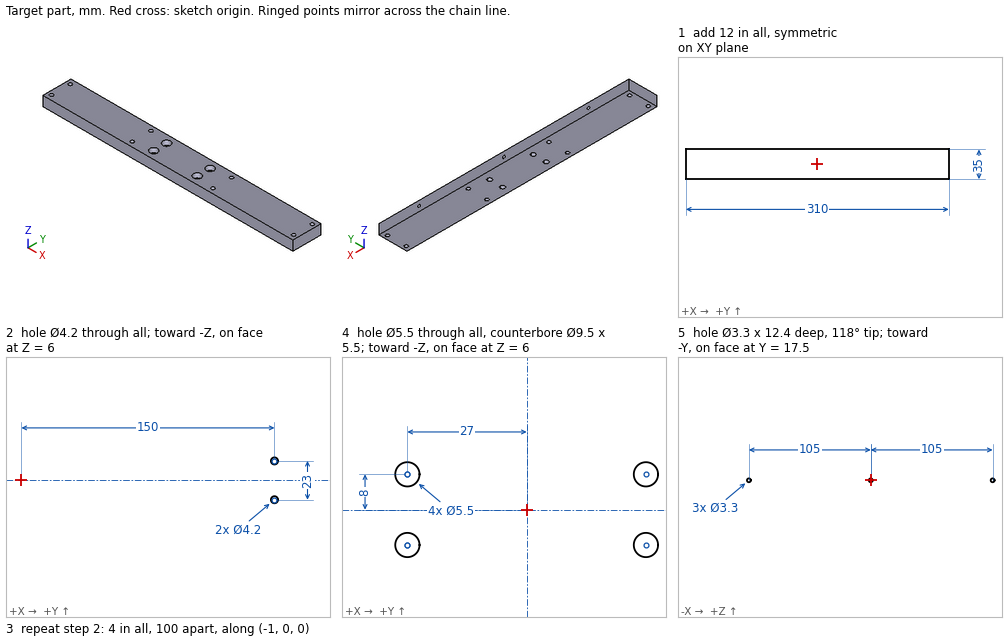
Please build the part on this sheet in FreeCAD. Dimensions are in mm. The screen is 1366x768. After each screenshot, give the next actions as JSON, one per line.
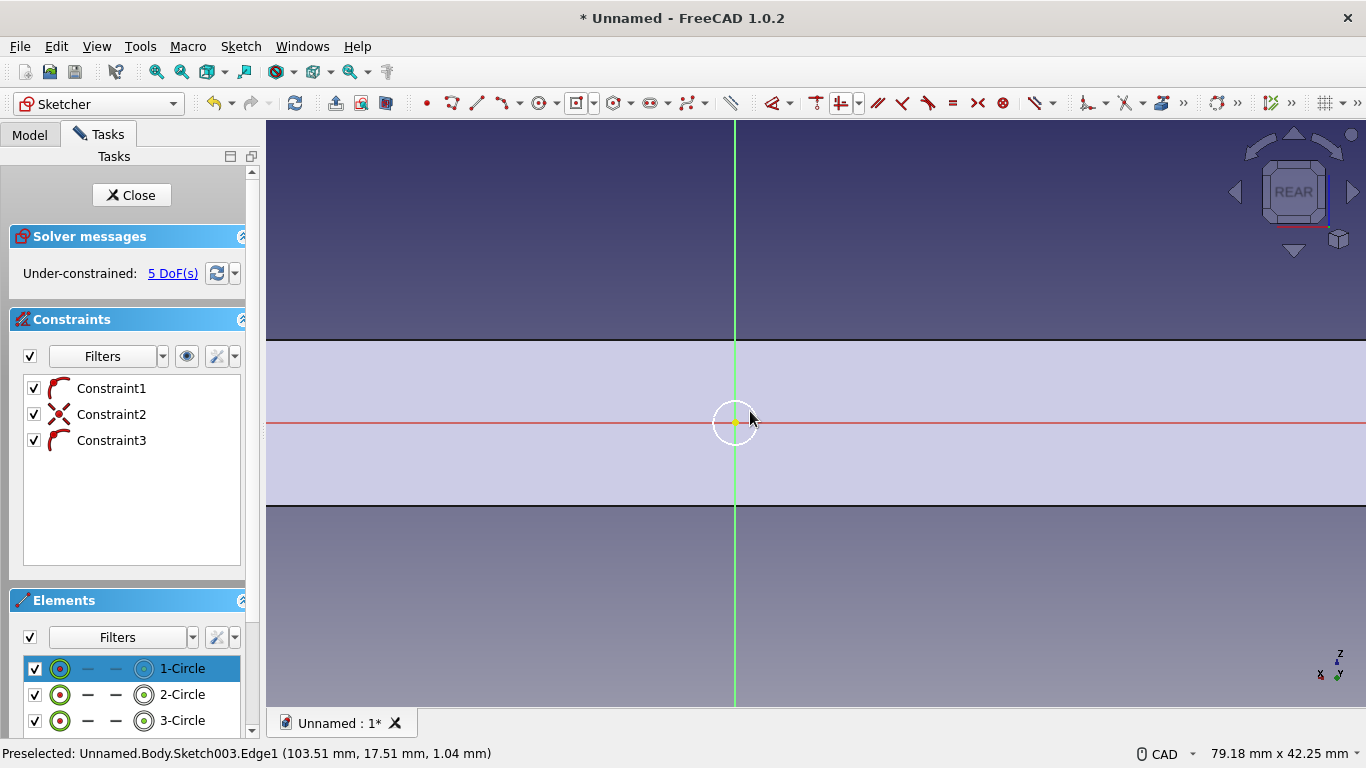
{"action": "left_click", "coordinate": [751, 407]}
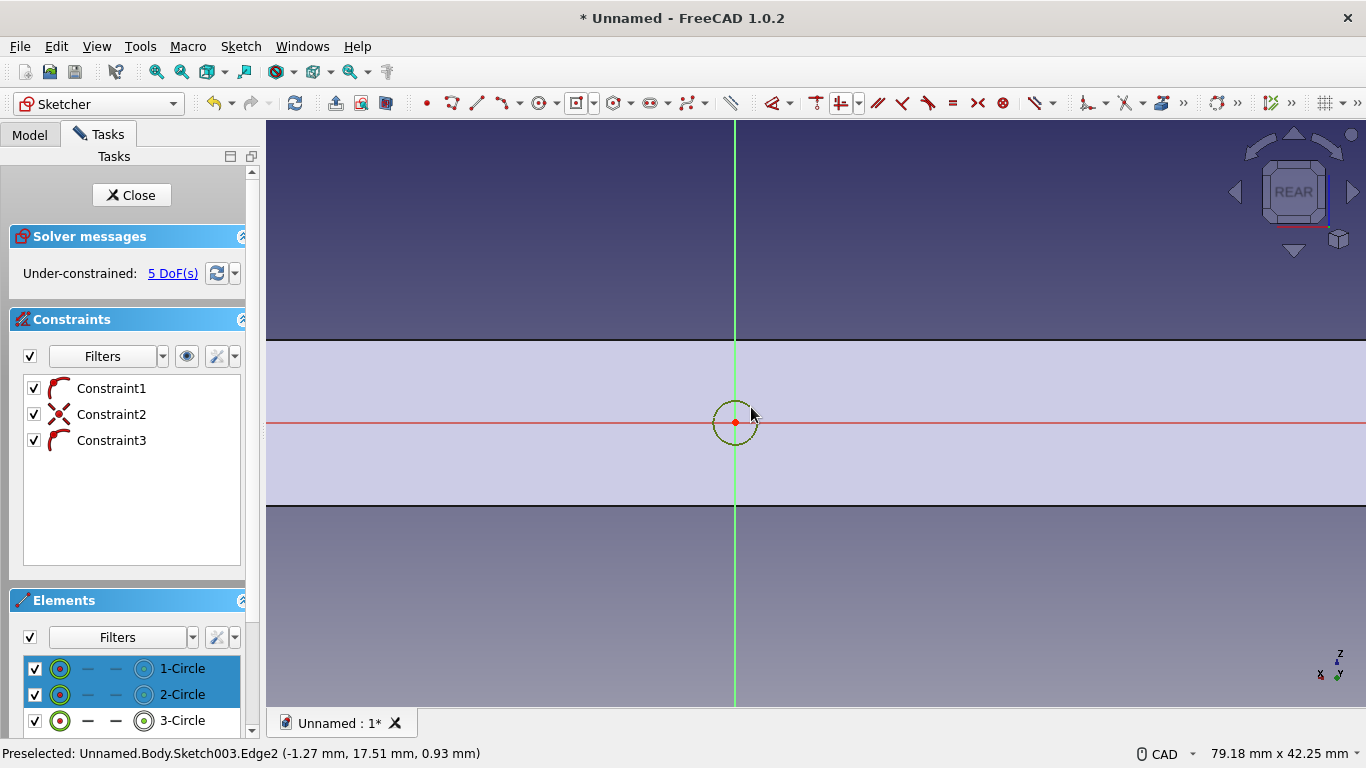
{"action": "scroll", "coordinate": [751, 411], "scroll_direction": "down", "scroll_amount": 8}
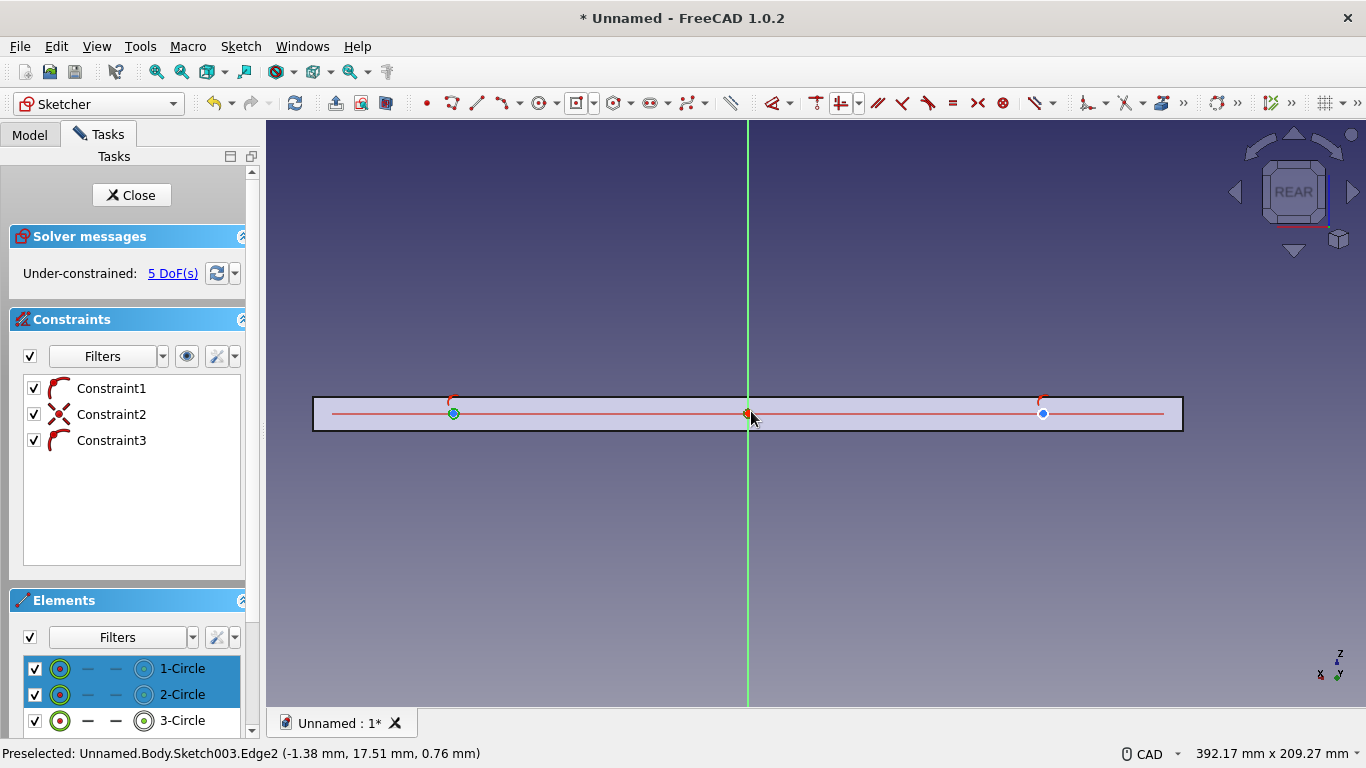
{"action": "scroll", "coordinate": [1047, 410], "scroll_direction": "up", "scroll_amount": 7}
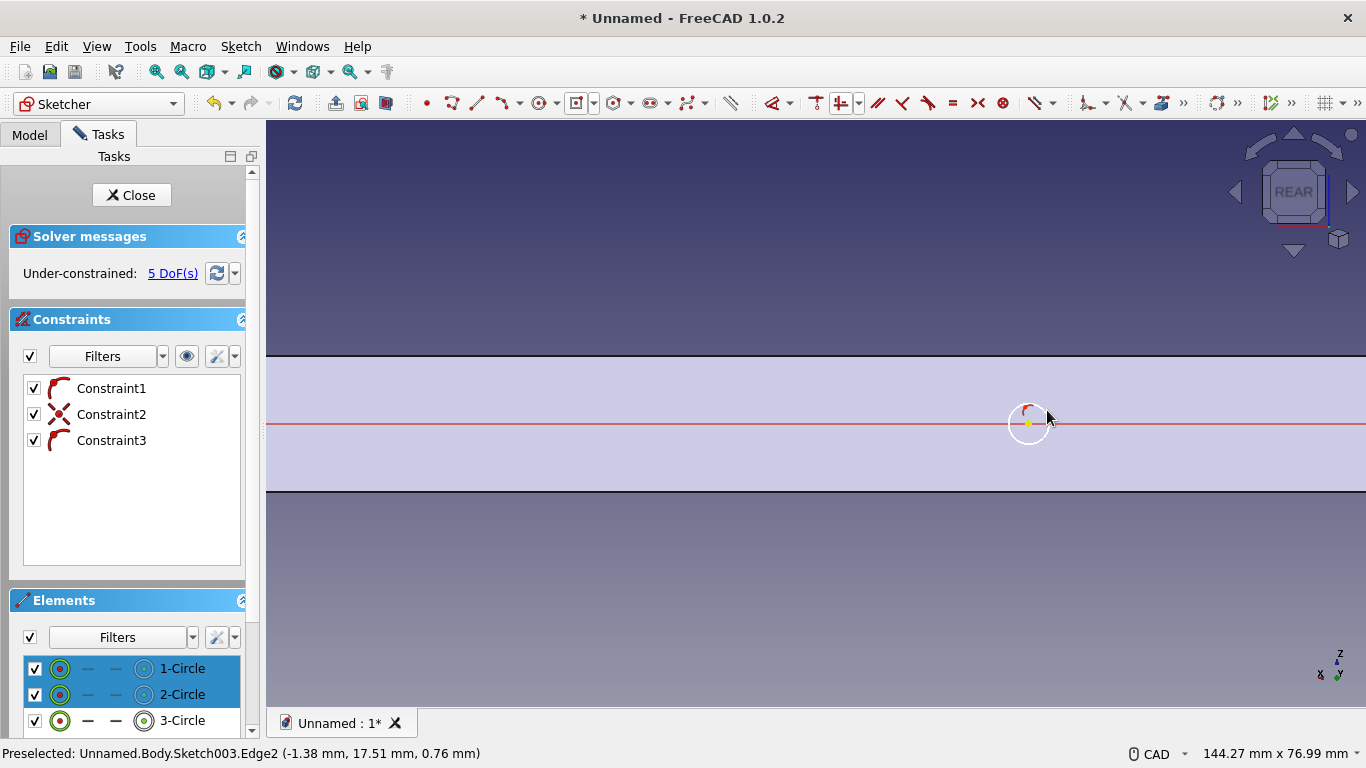
{"action": "left_click", "coordinate": [1043, 410]}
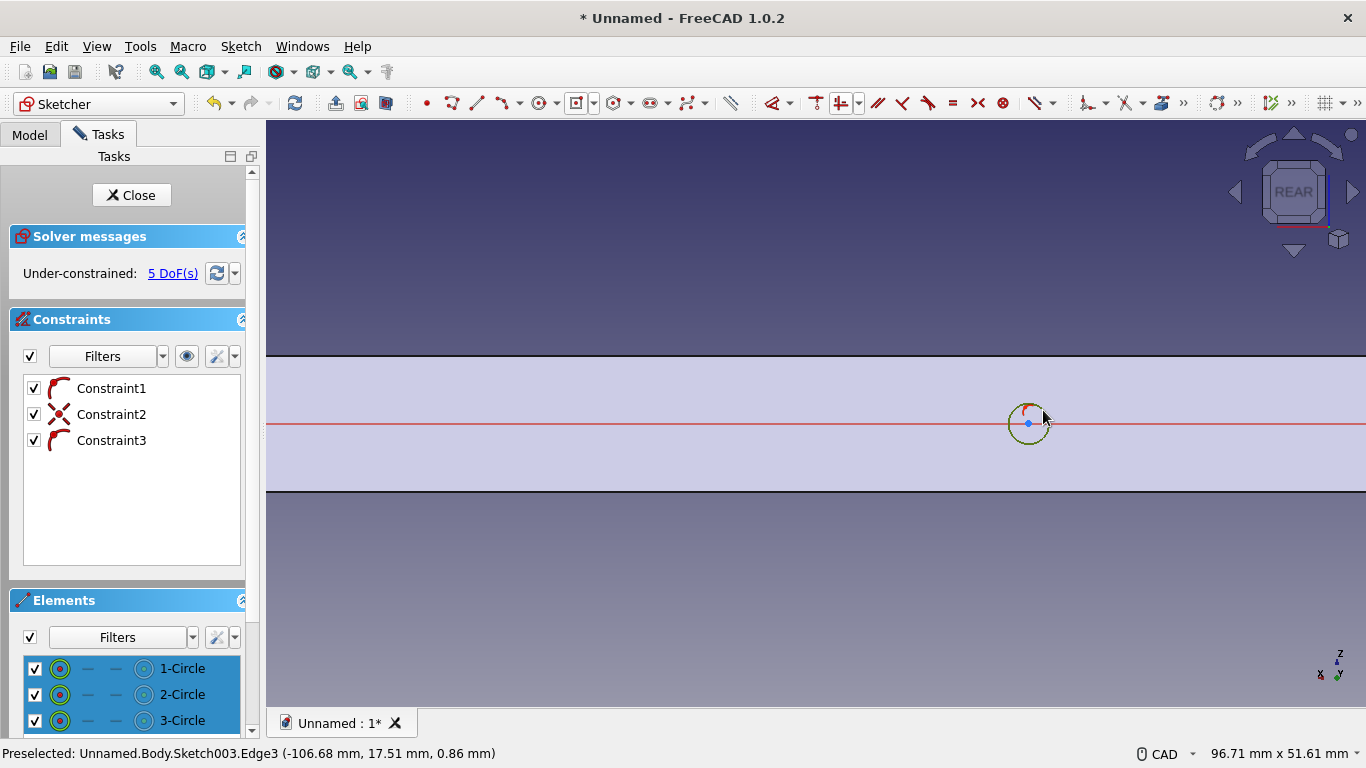
{"action": "left_click", "coordinate": [953, 104]}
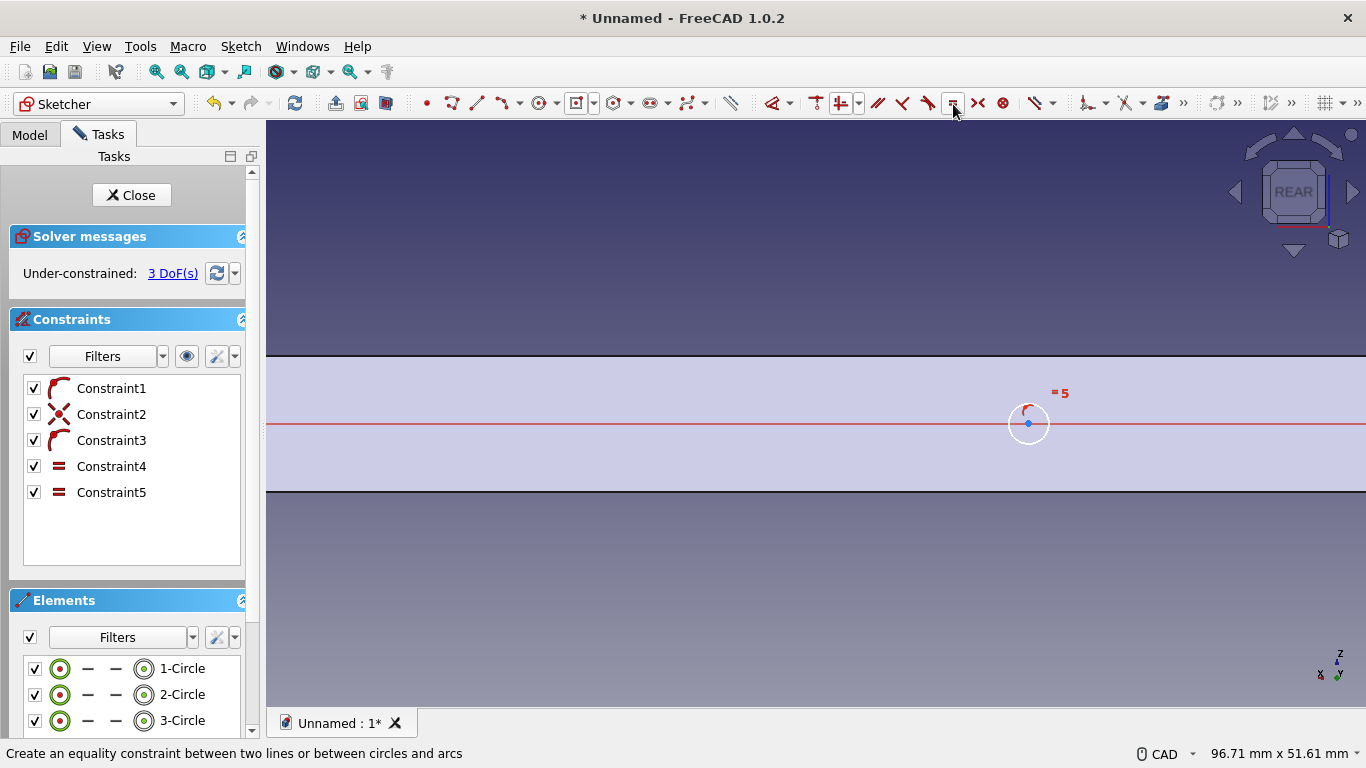
{"action": "left_click", "coordinate": [772, 104]}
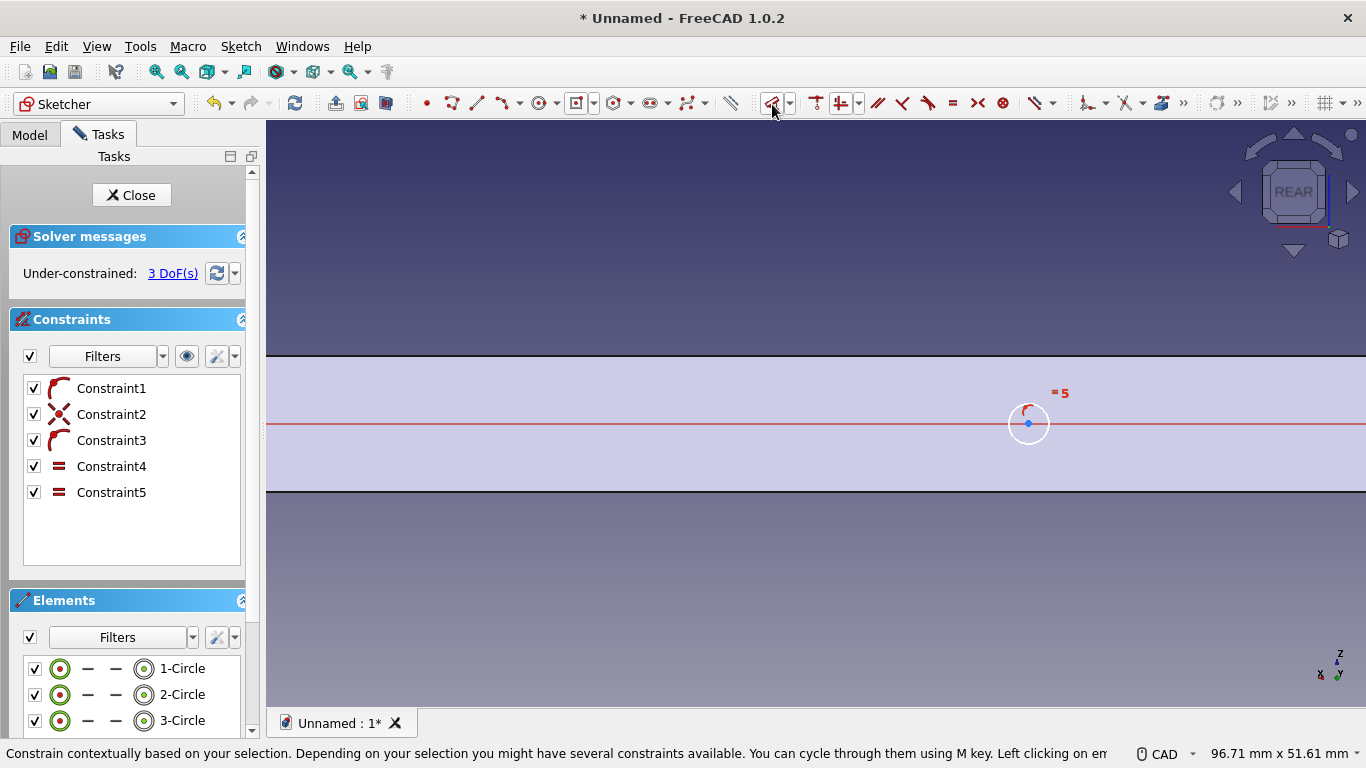
{"action": "scroll", "coordinate": [1047, 410], "scroll_direction": "down", "scroll_amount": 7}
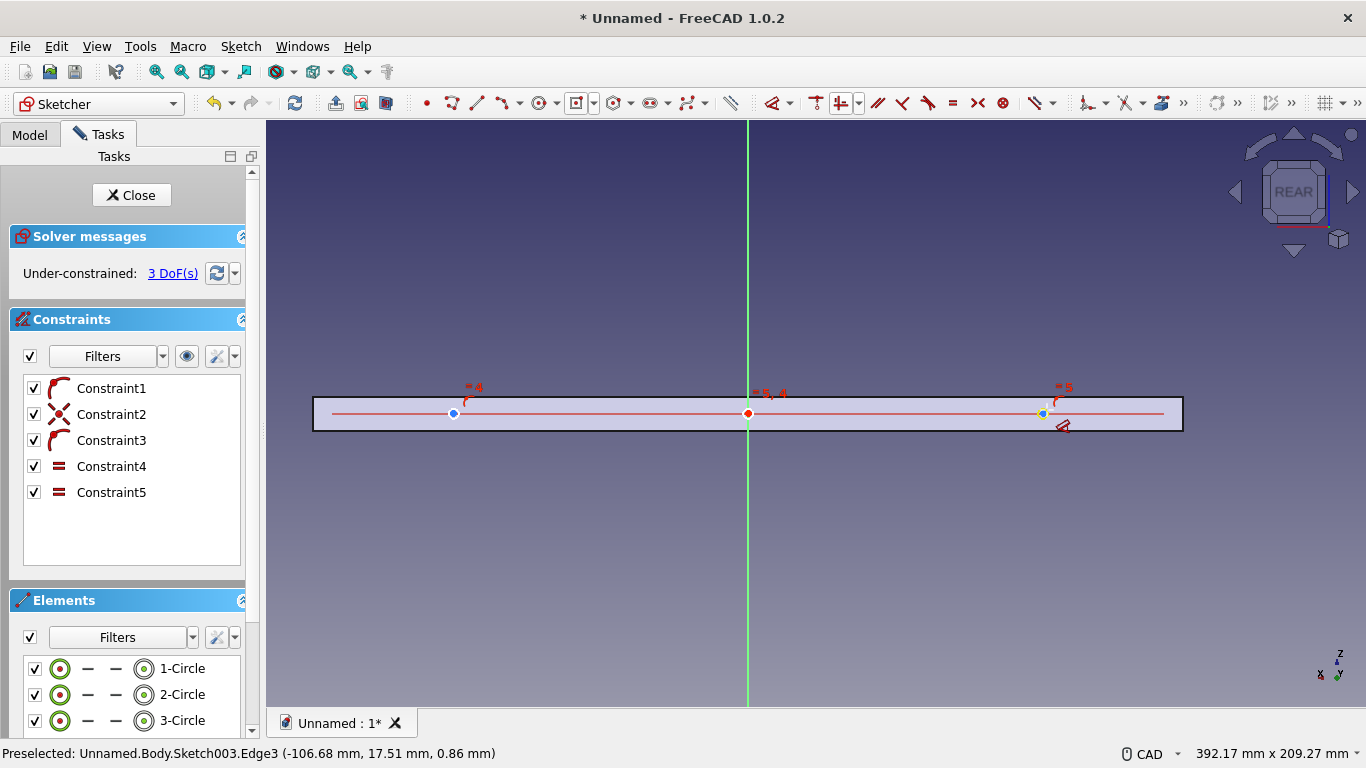
{"action": "scroll", "coordinate": [457, 410], "scroll_direction": "up", "scroll_amount": 8}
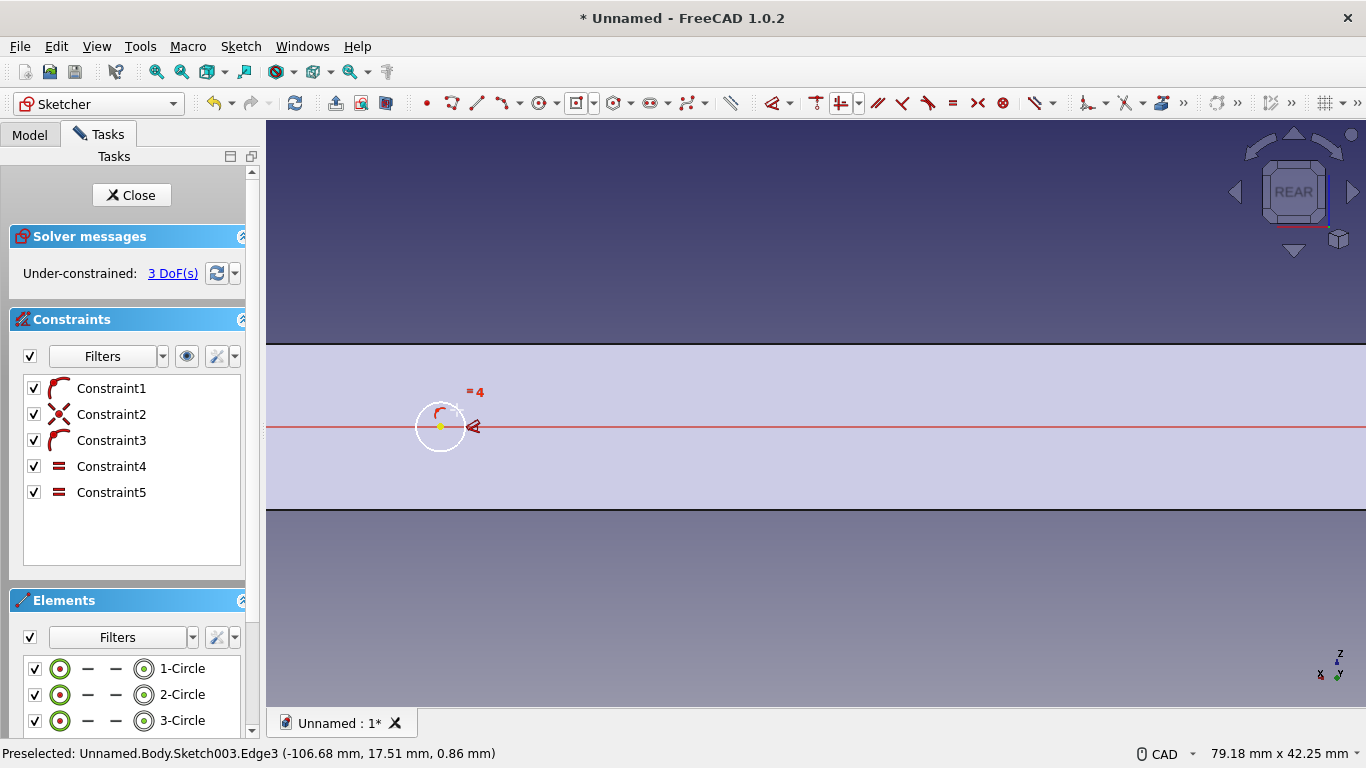
{"action": "left_click", "coordinate": [458, 410]}
{"action": "left_click", "coordinate": [481, 388]}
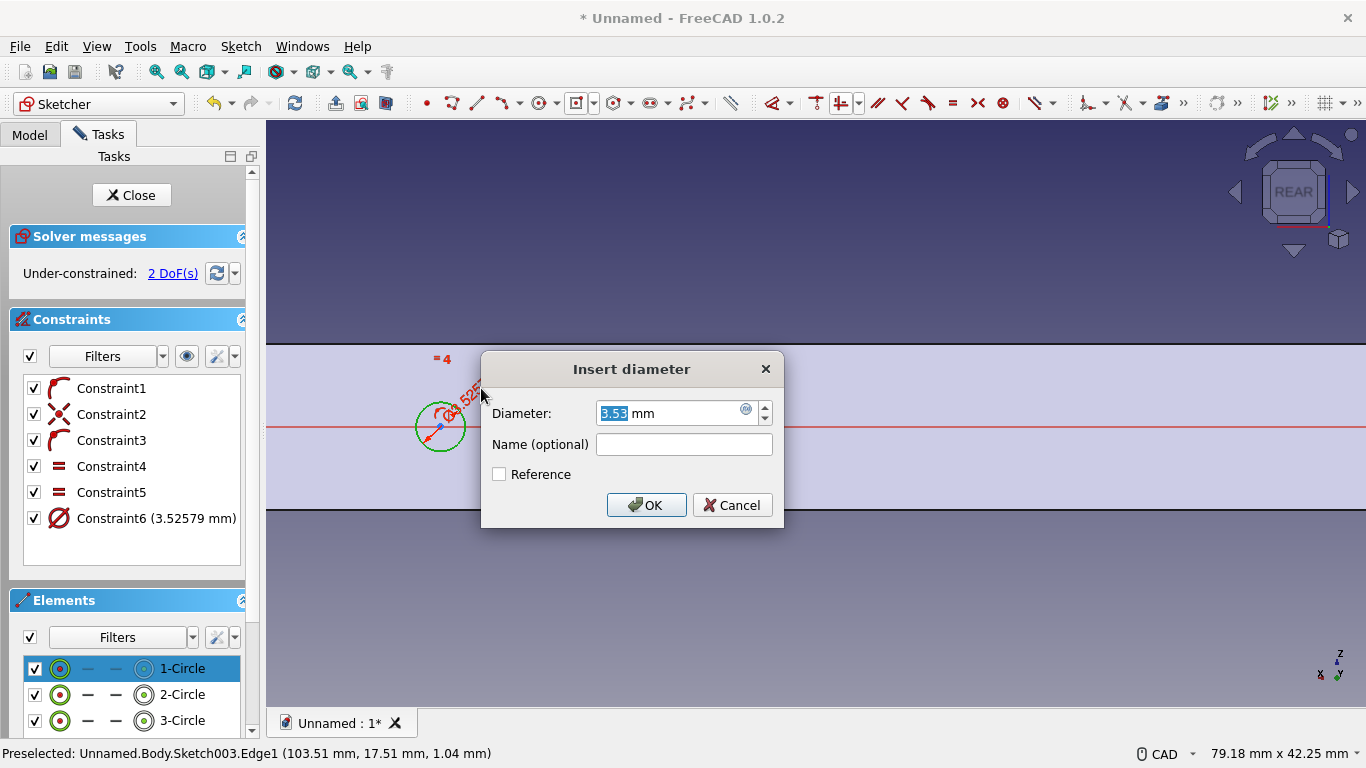
{"action": "type", "text": "3.3"}
{"action": "key", "text": "Return"}